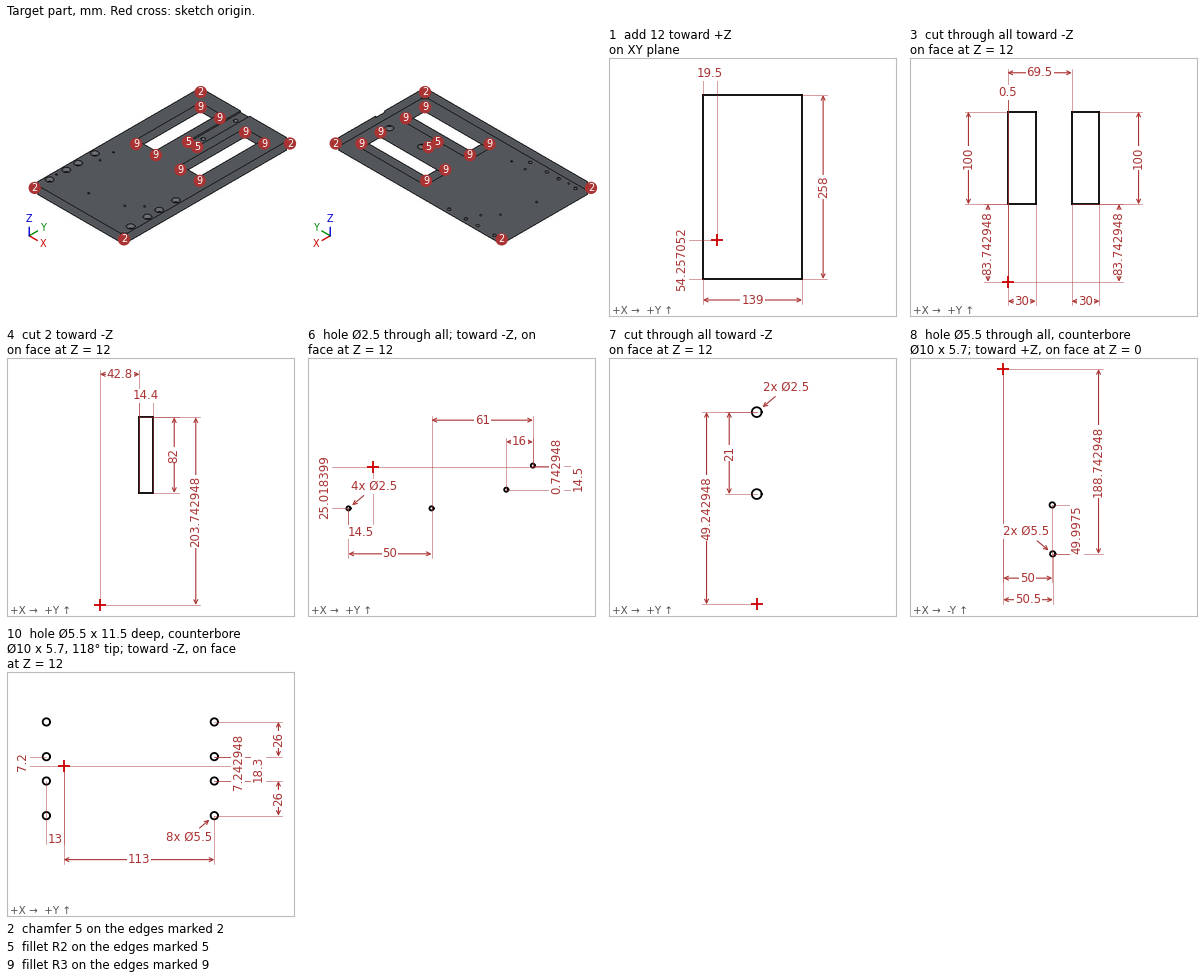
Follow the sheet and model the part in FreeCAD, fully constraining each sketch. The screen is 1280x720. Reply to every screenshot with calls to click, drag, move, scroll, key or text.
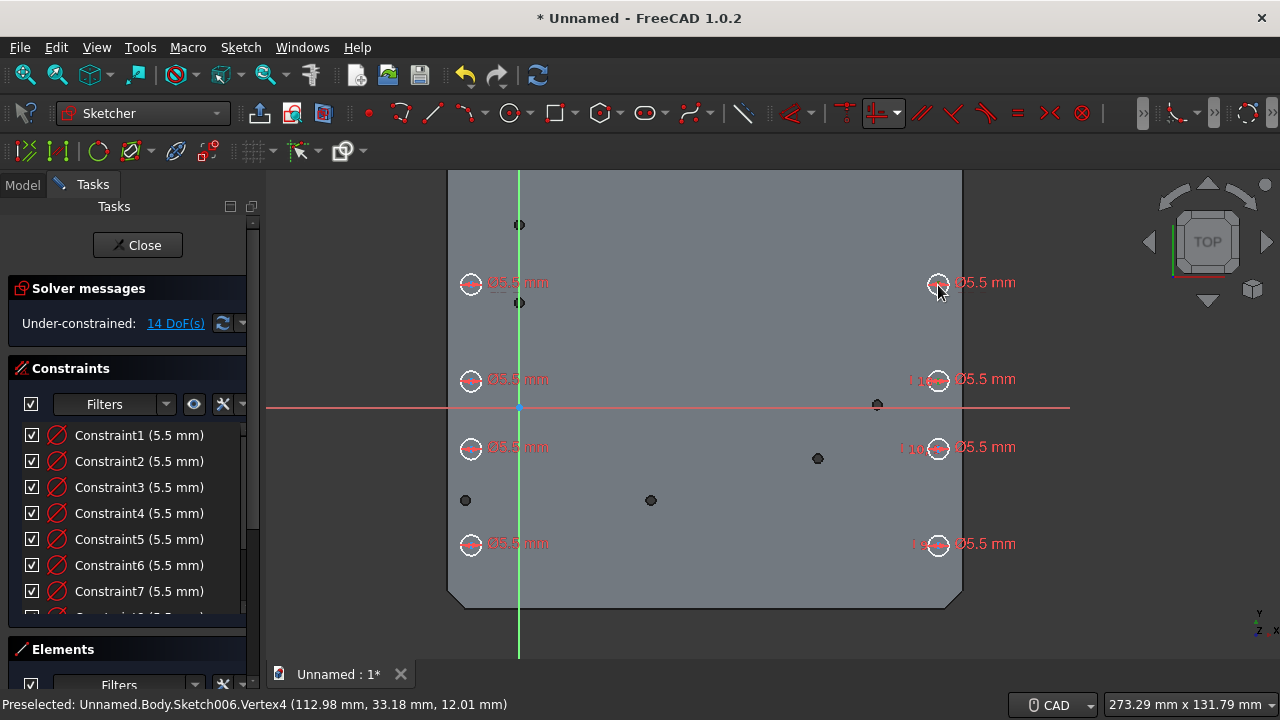
key(v)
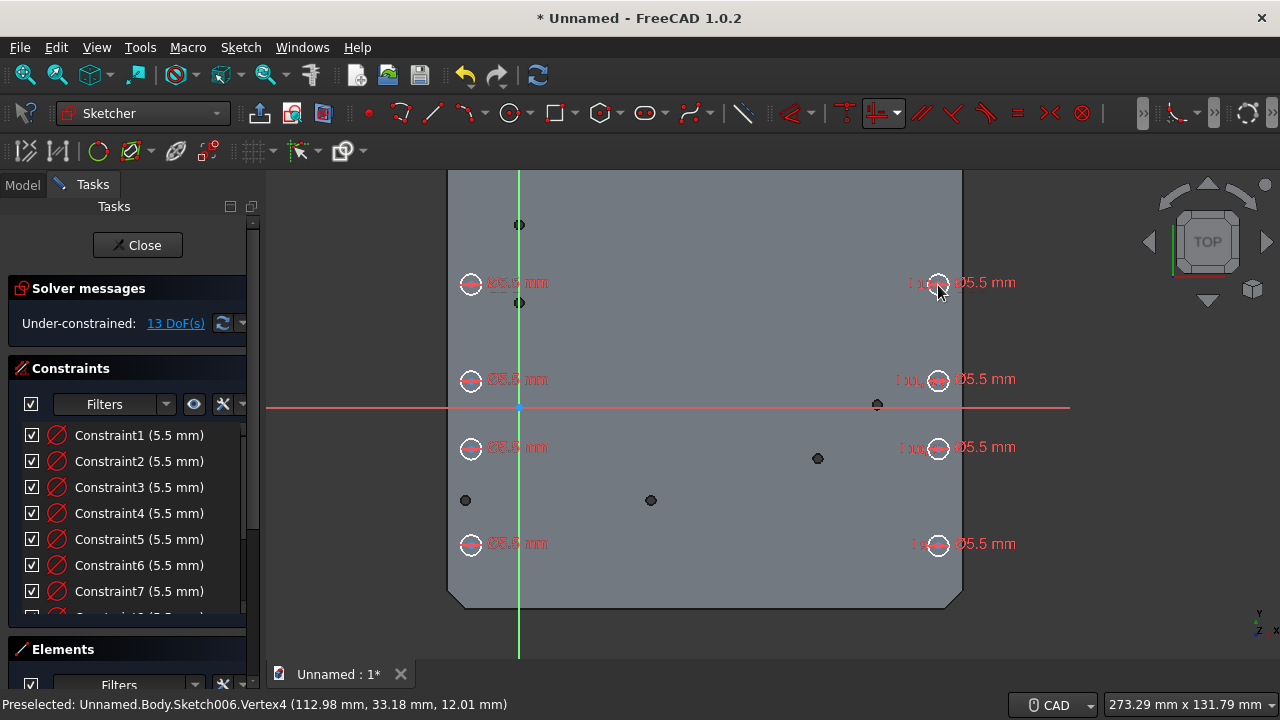
click(938, 449)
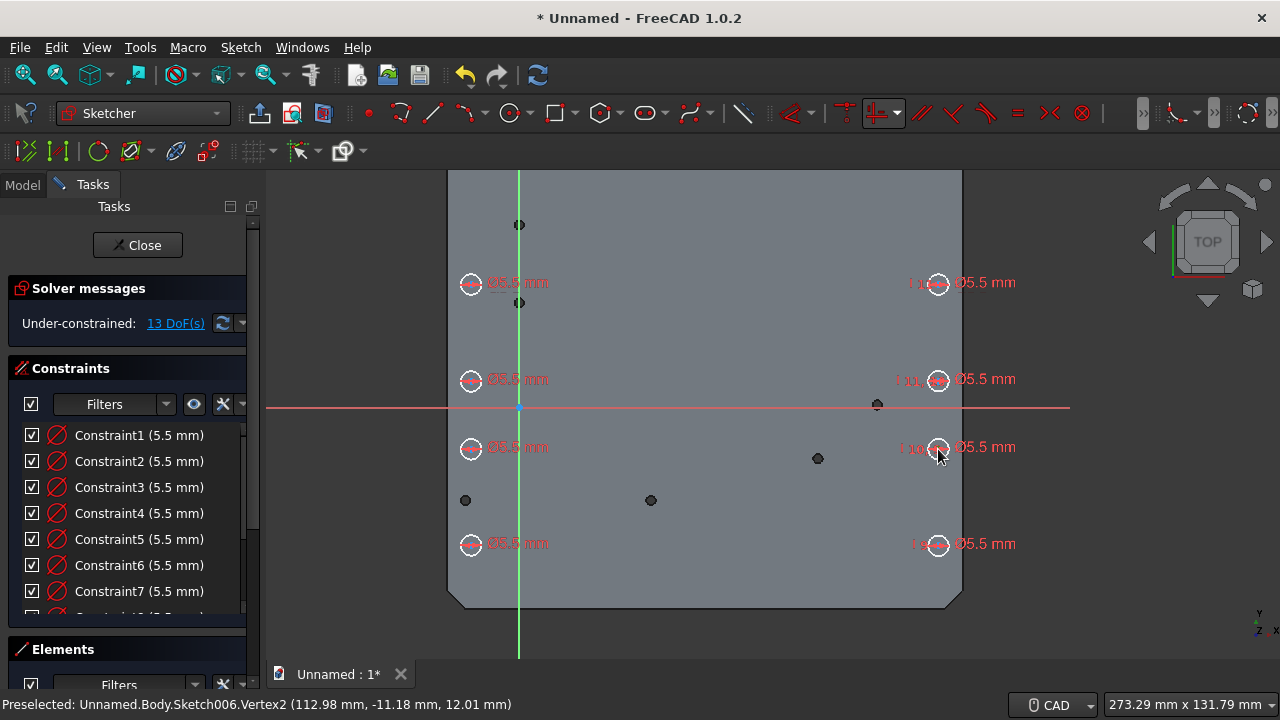
click(471, 449)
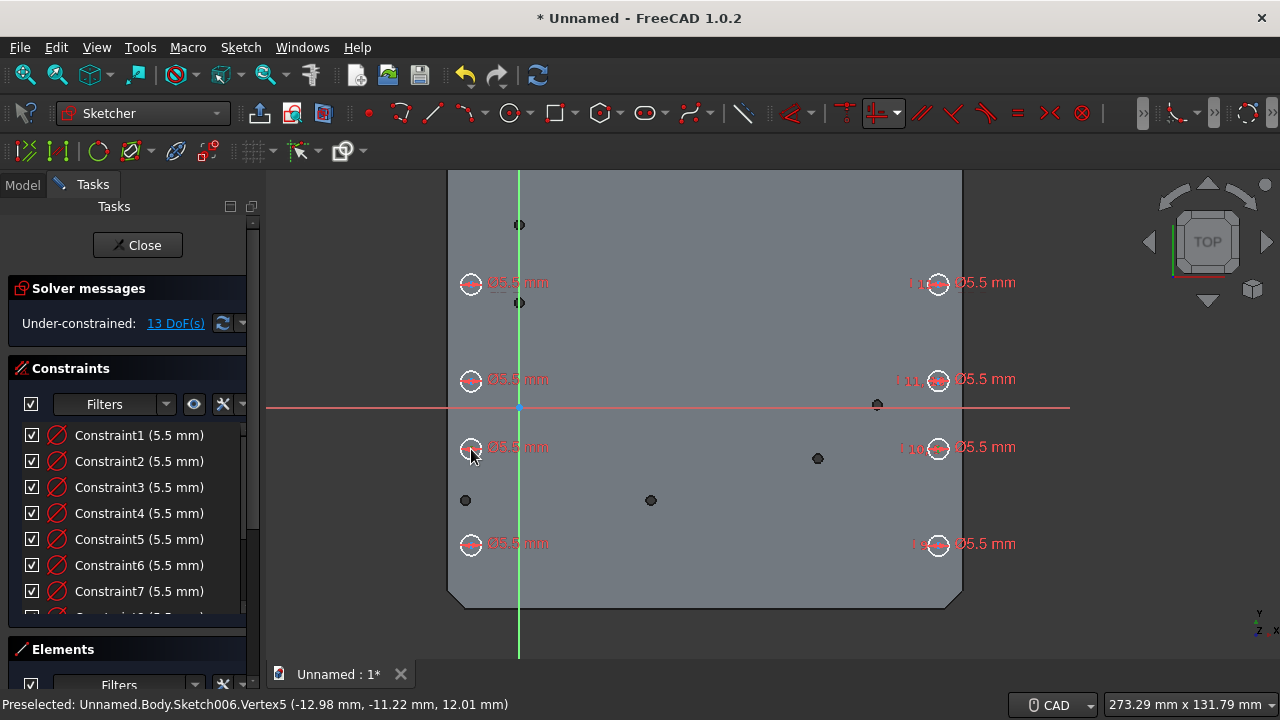
key(h)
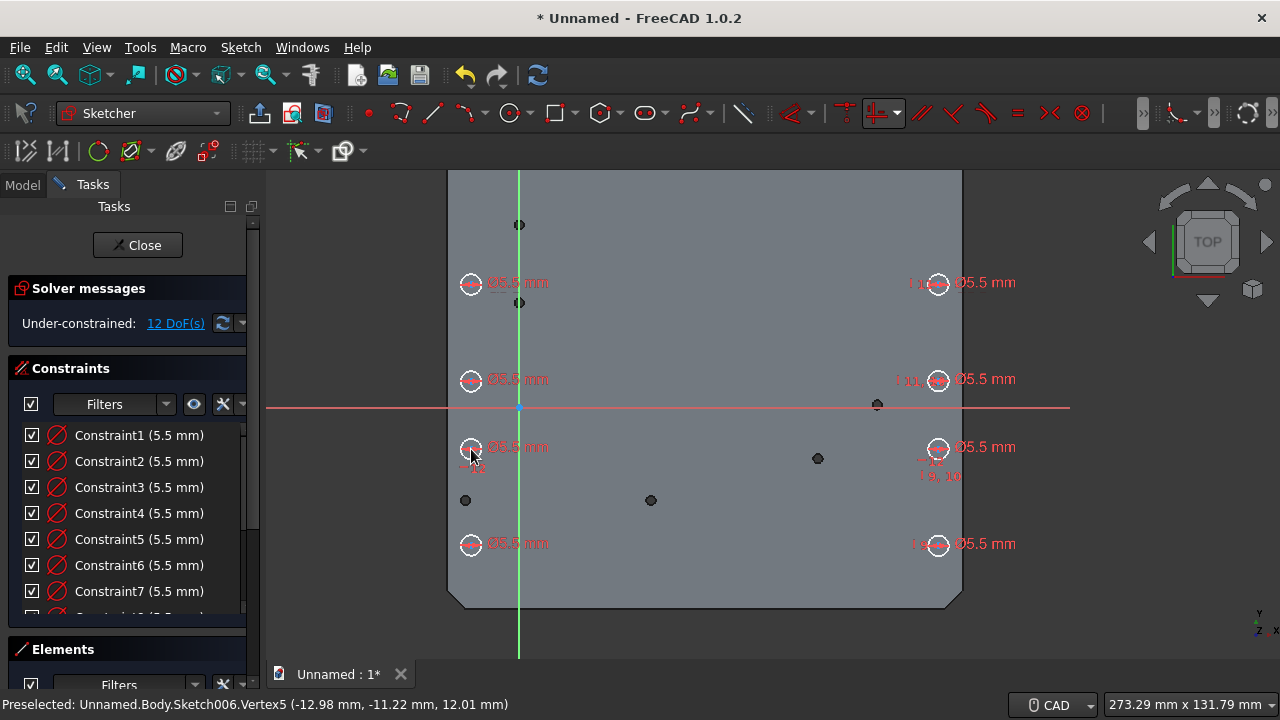
click(471, 449)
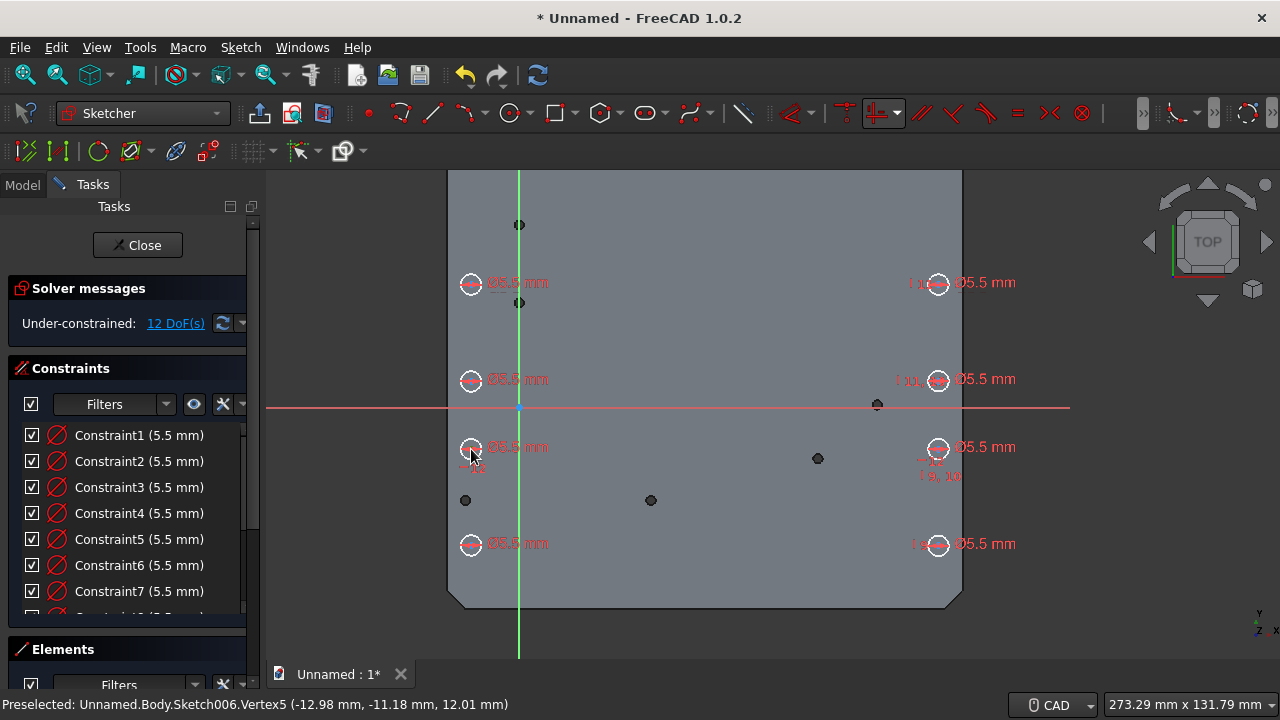
click(471, 381)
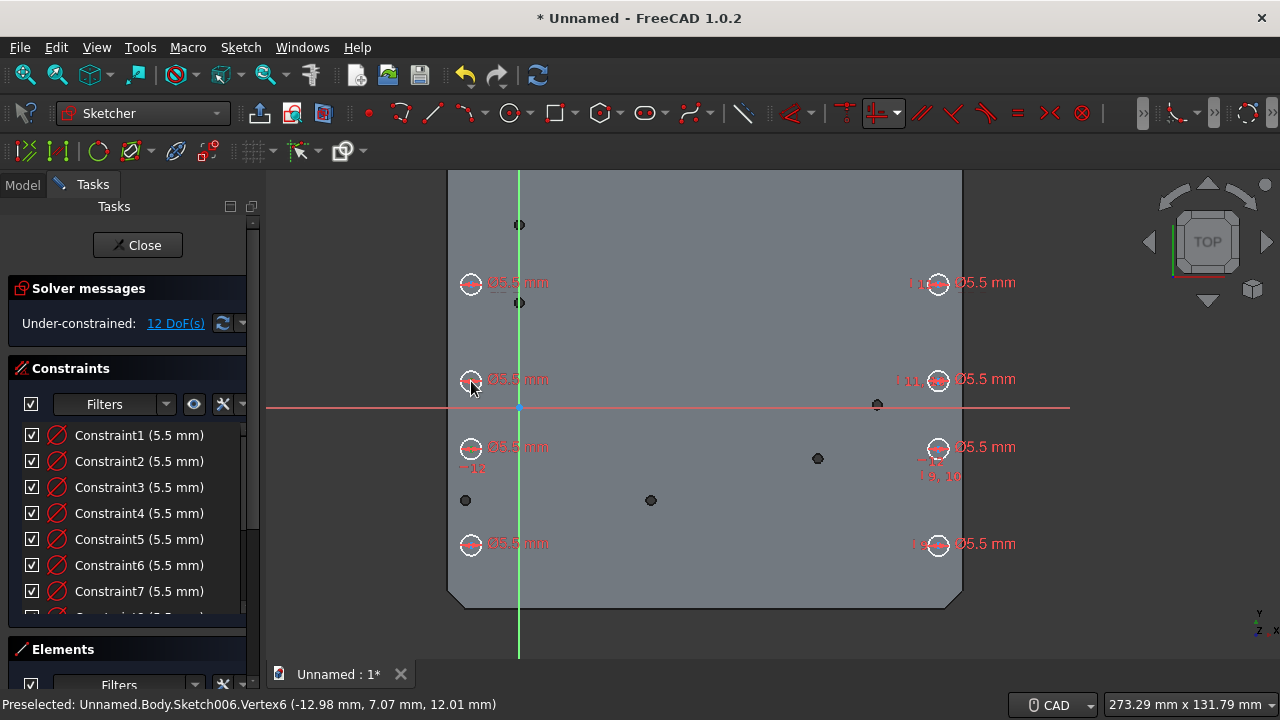
key(v)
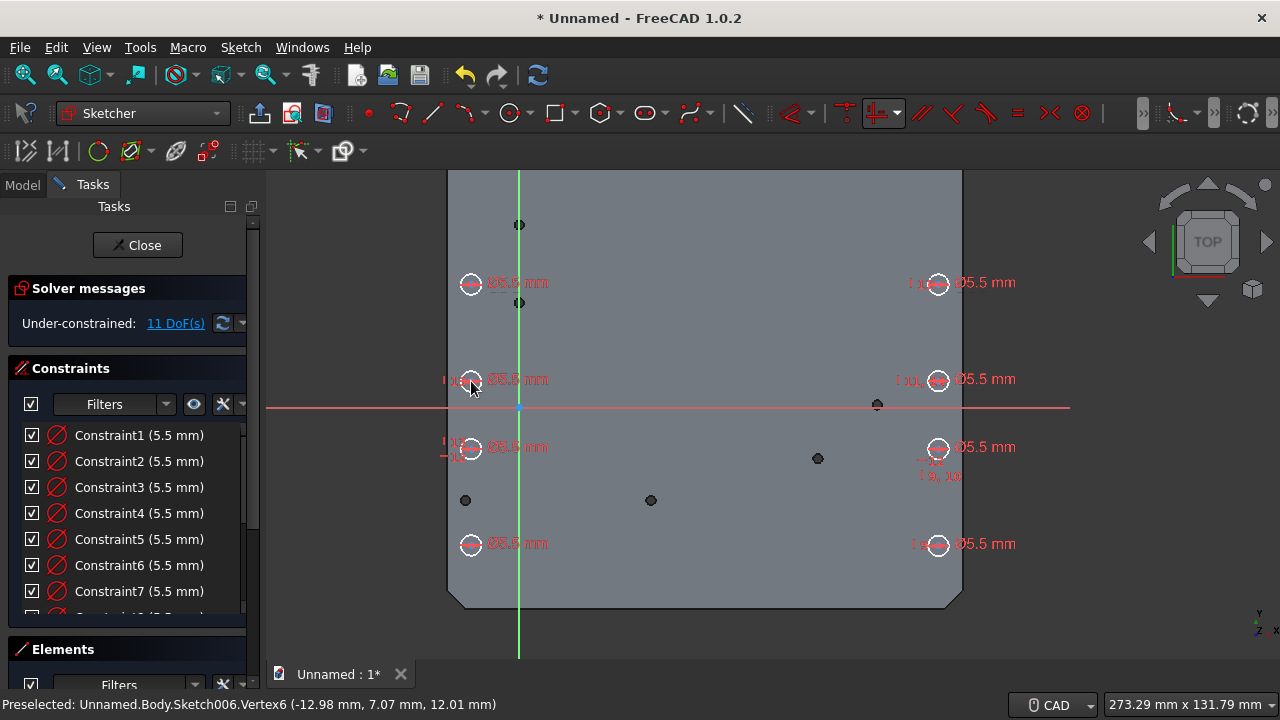
click(471, 449)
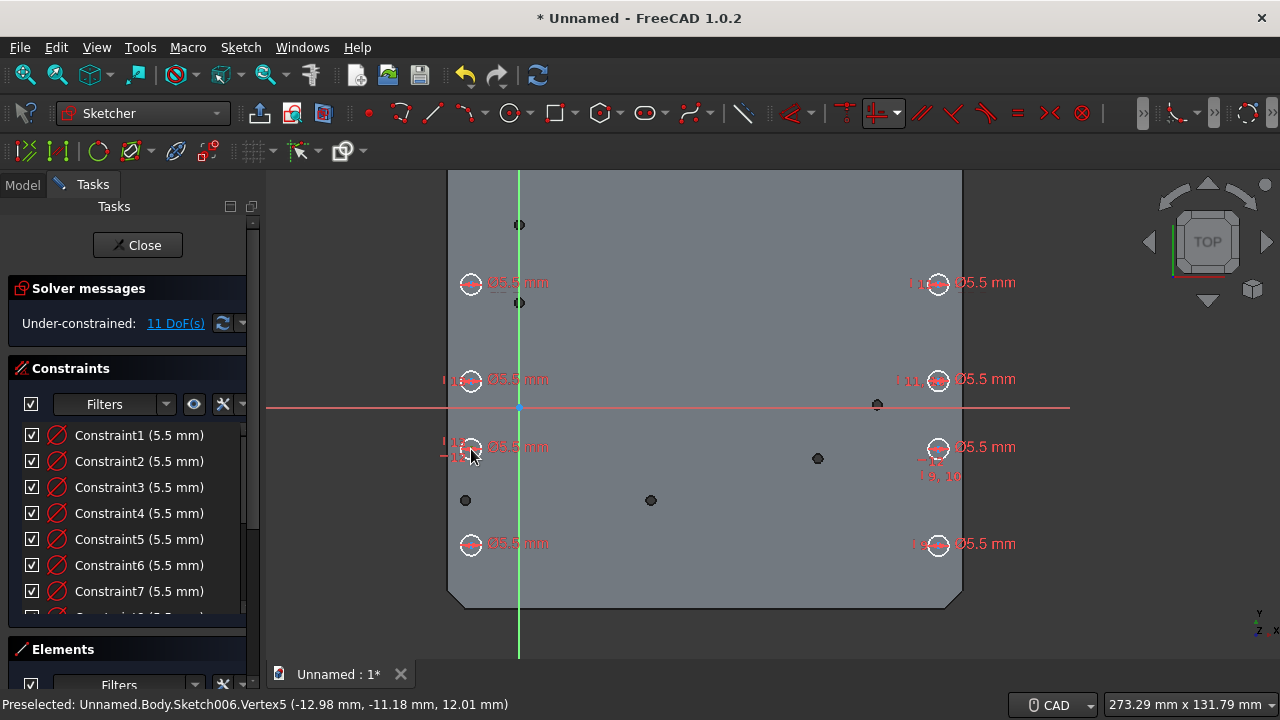
click(471, 545)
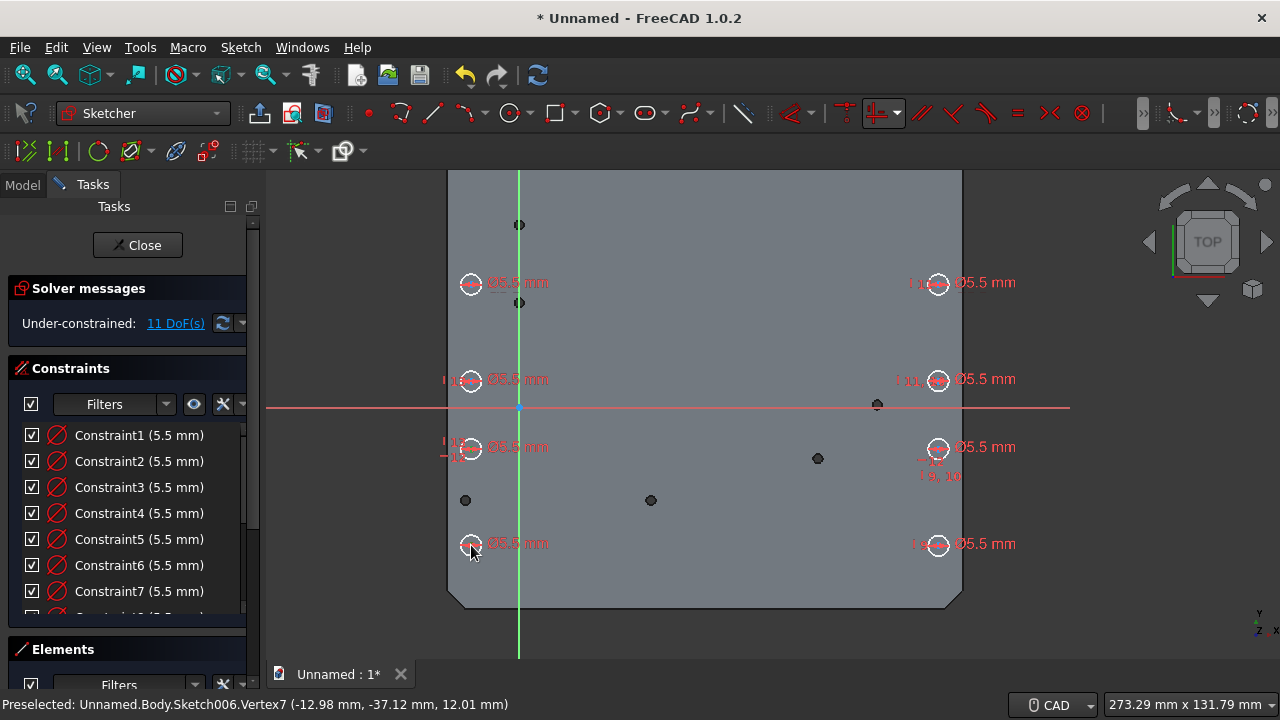
key(v)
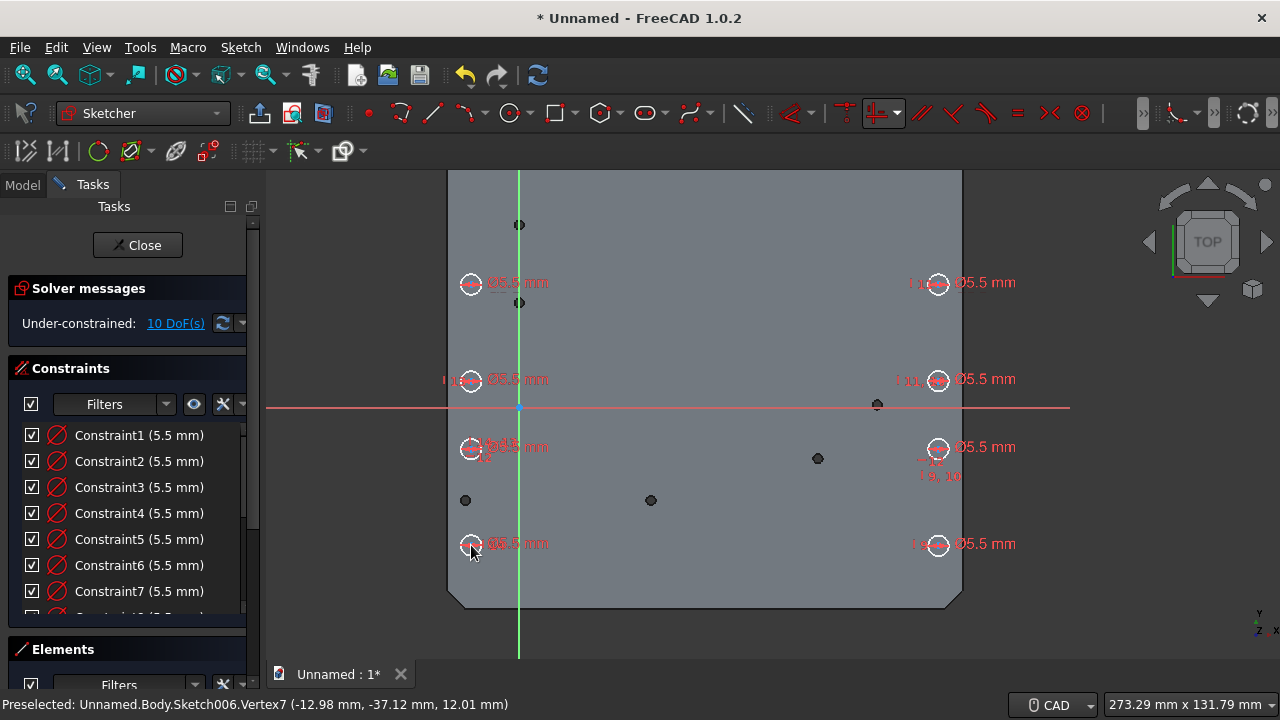
click(938, 546)